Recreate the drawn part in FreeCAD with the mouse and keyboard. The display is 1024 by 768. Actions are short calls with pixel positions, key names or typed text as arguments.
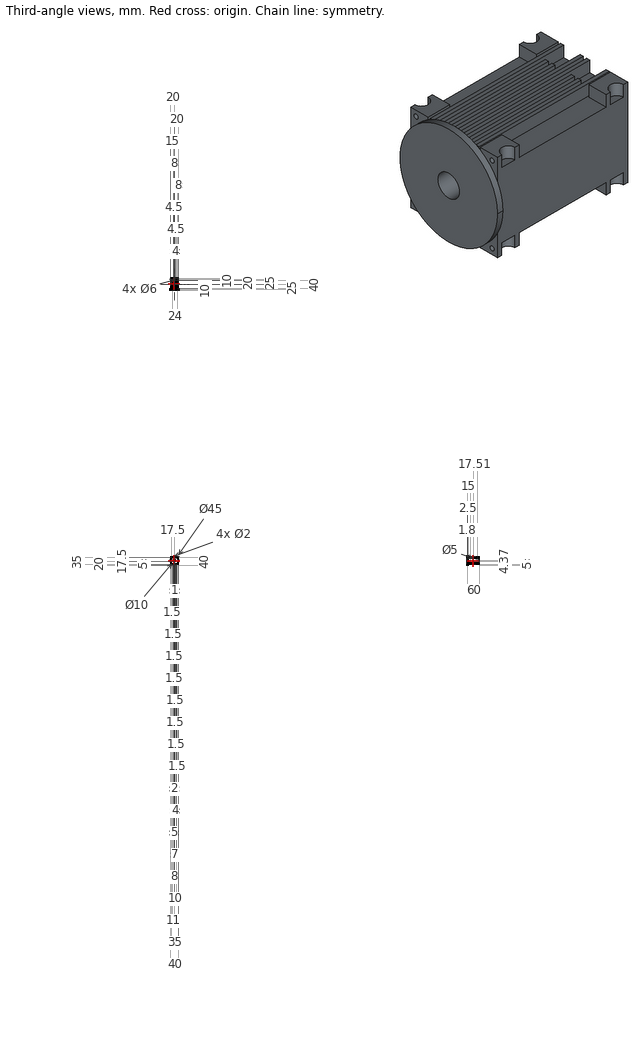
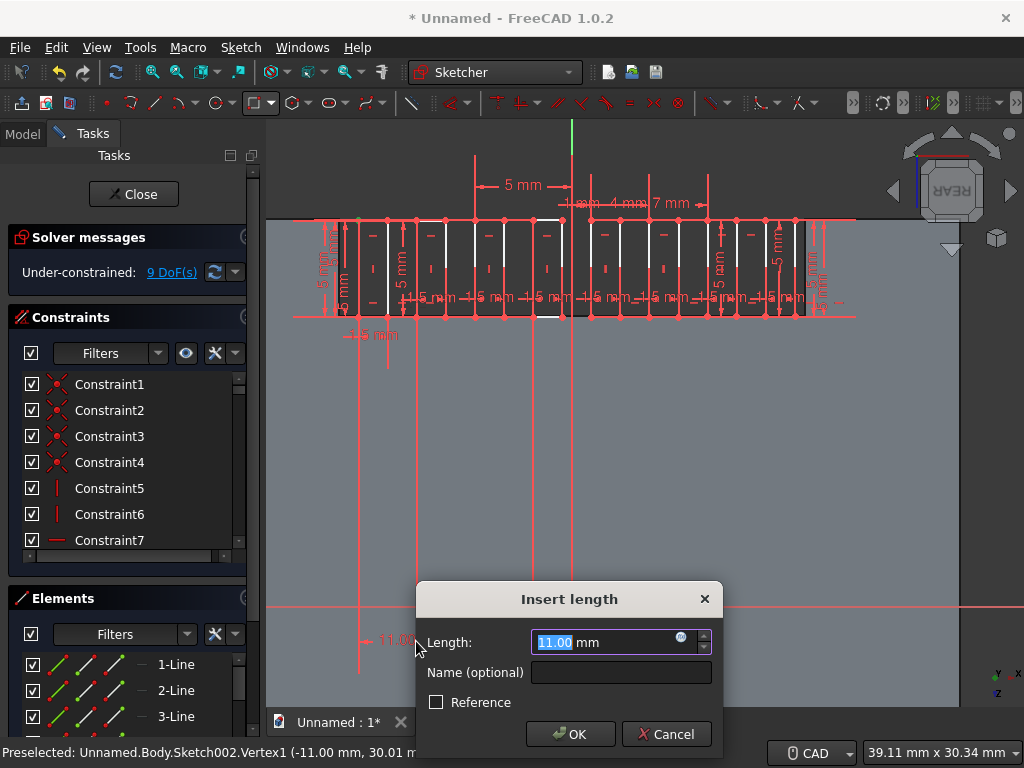
text(11)
key(Return)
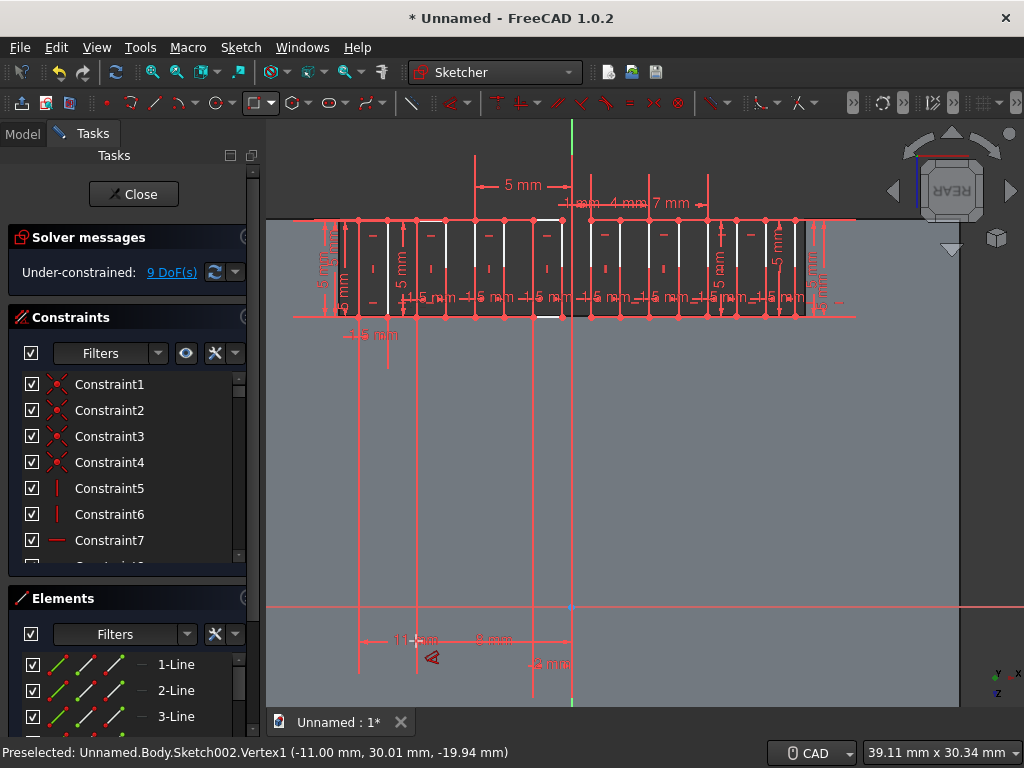
click(359, 221)
click(325, 414)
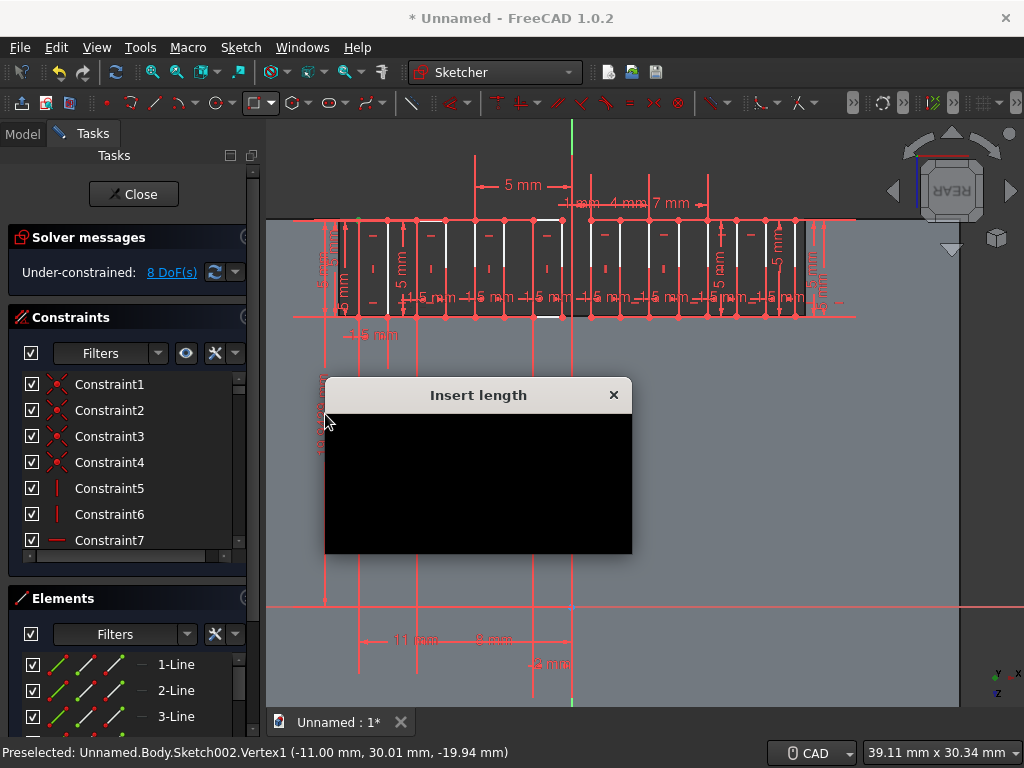
text(20)
key(Return)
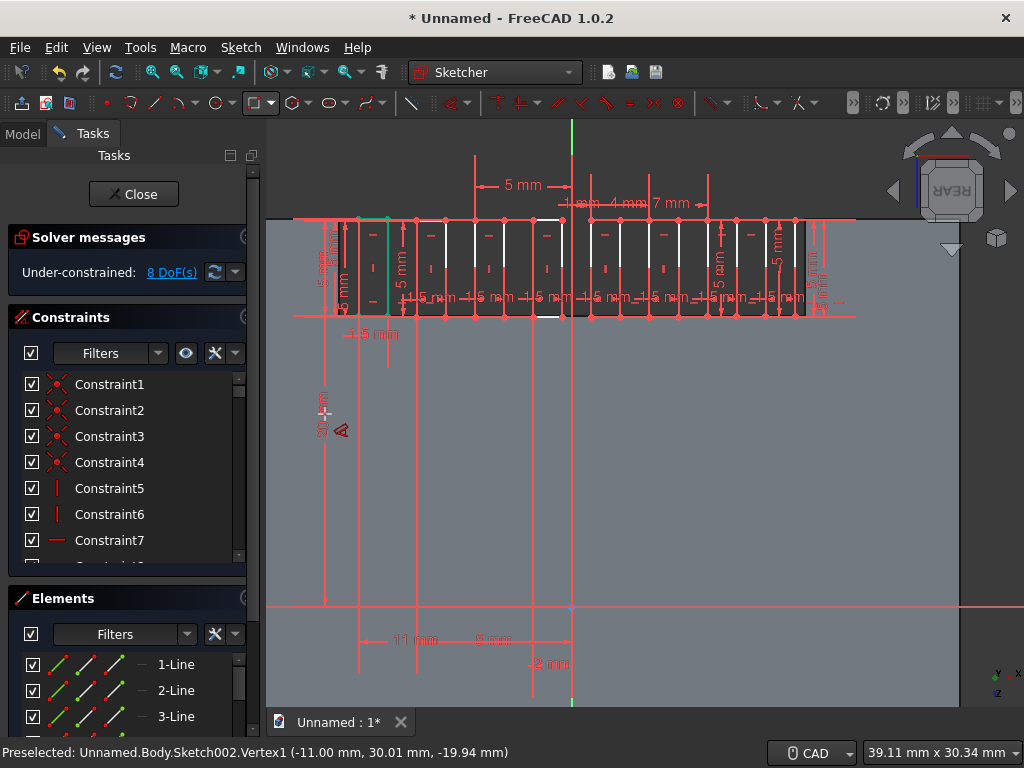
click(417, 221)
click(383, 503)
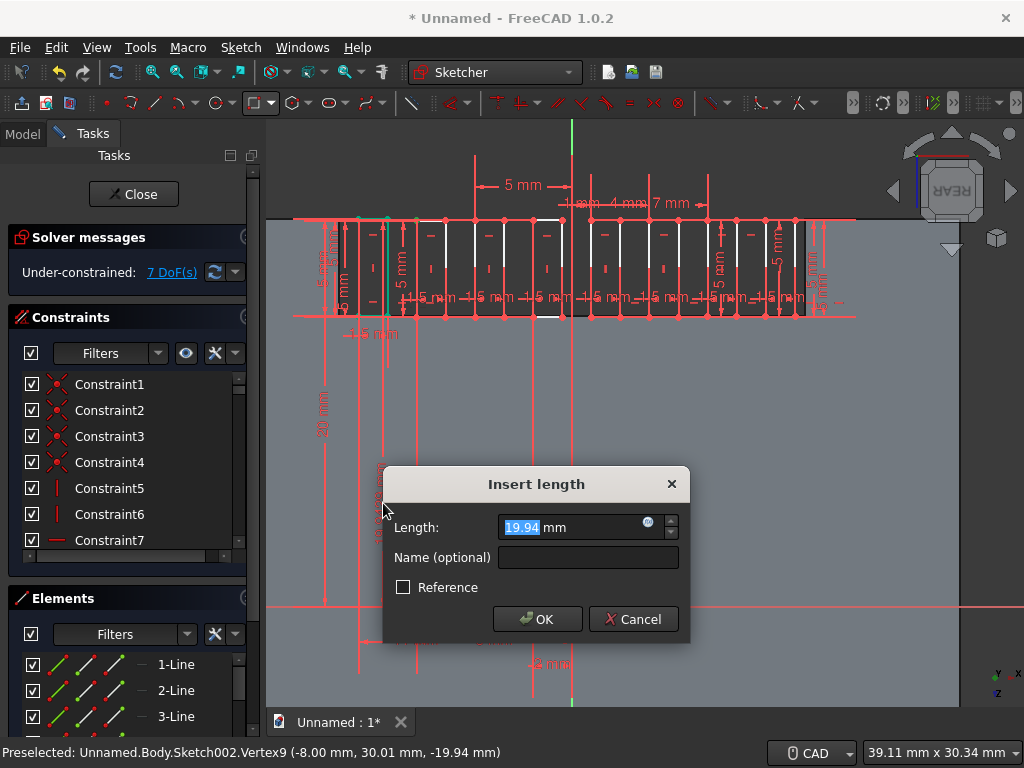
text(20)
key(Return)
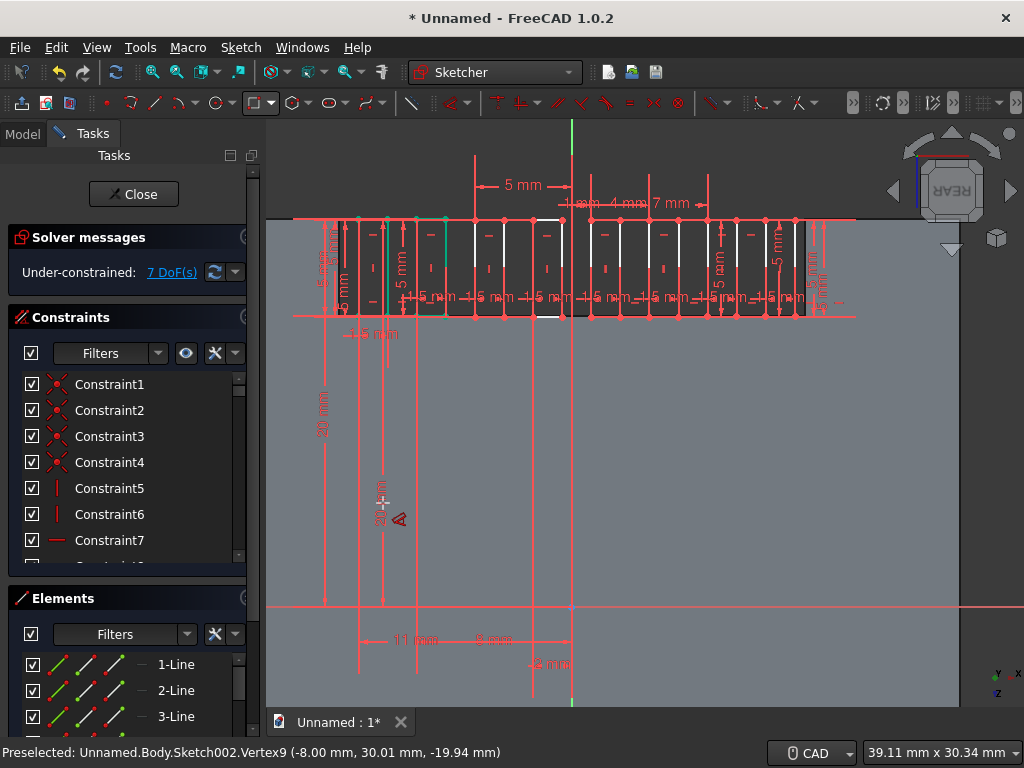
click(475, 220)
click(441, 414)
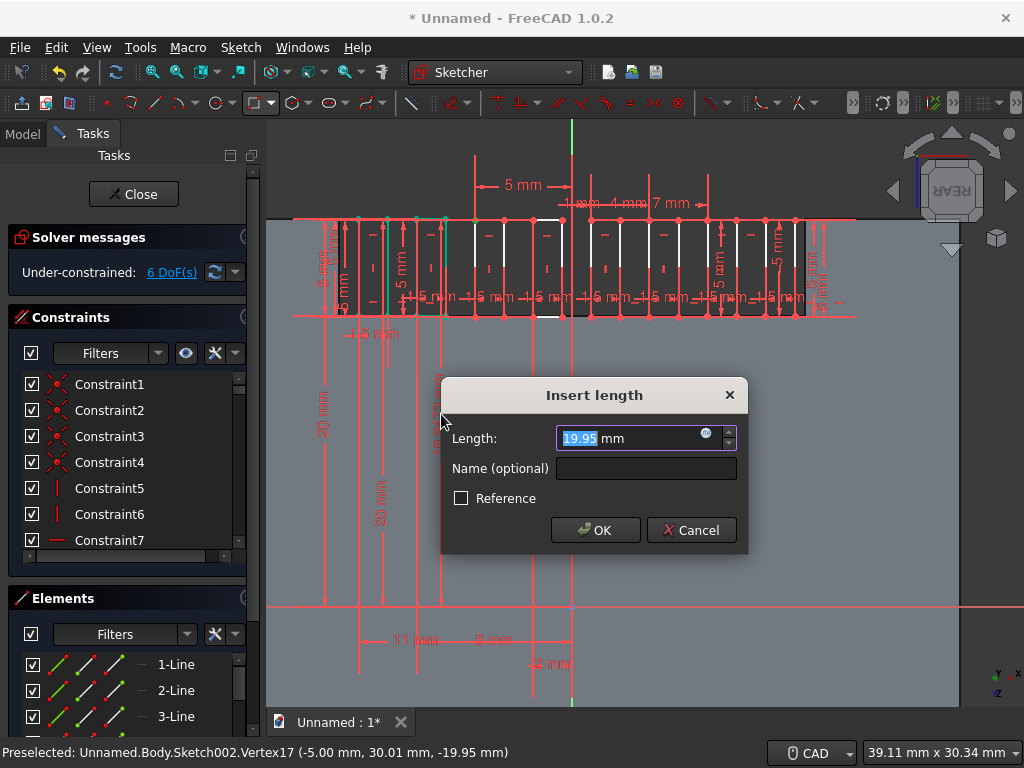
text(20)
key(Return)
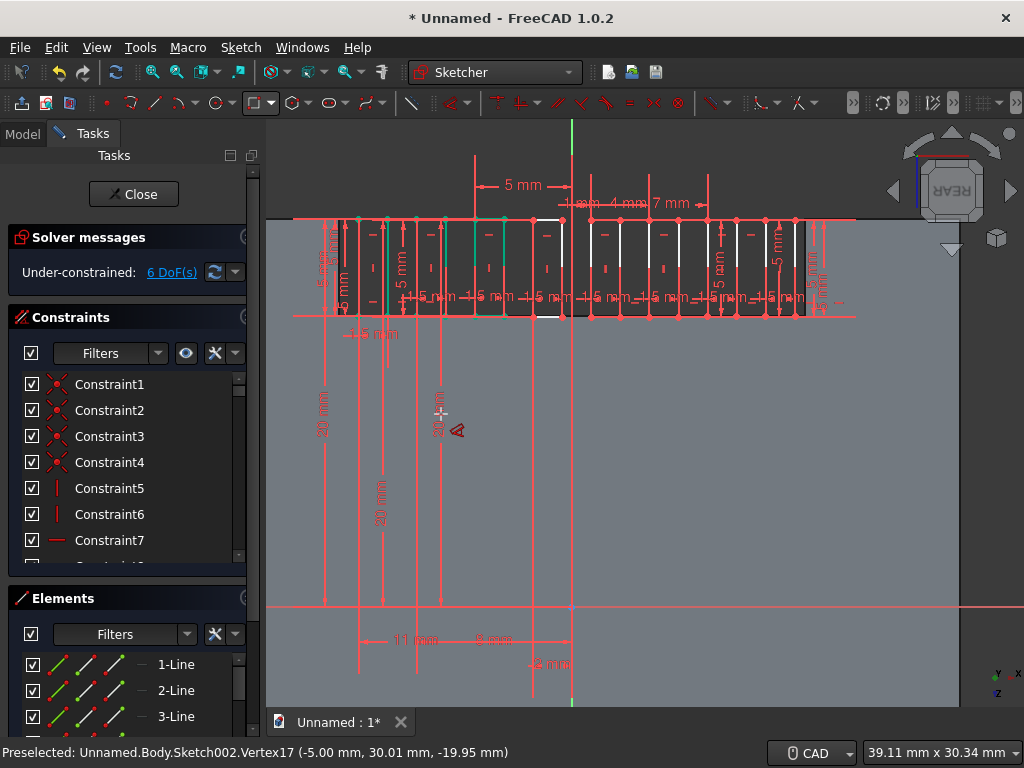
click(533, 220)
click(499, 503)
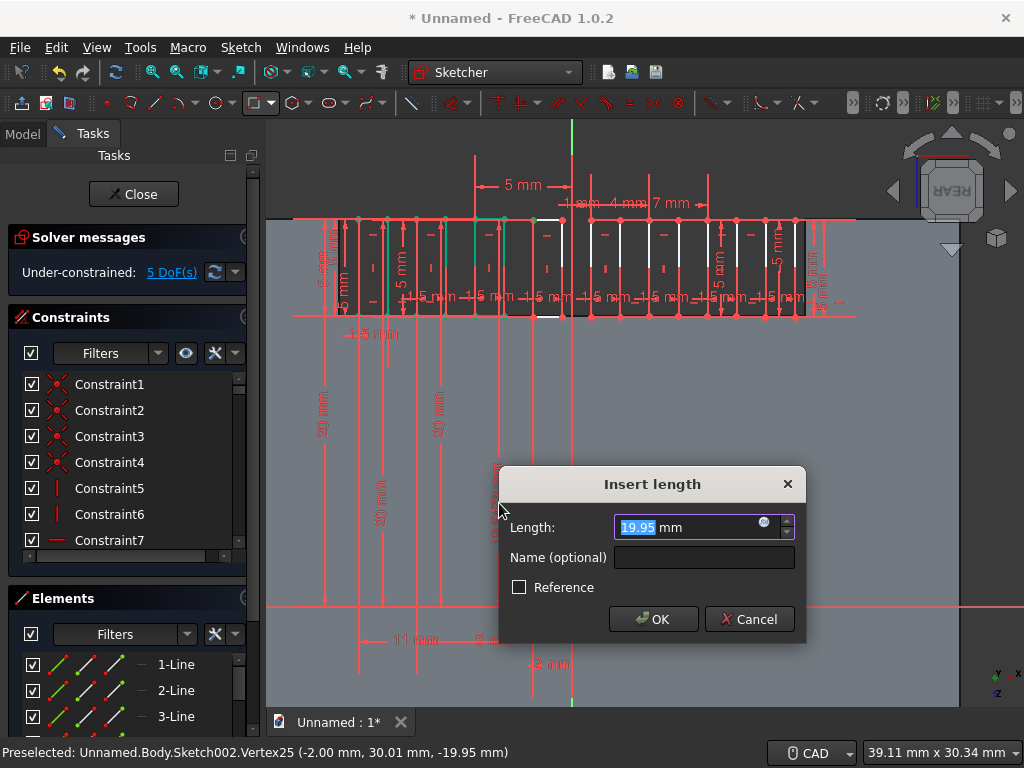
text(20)
key(Return)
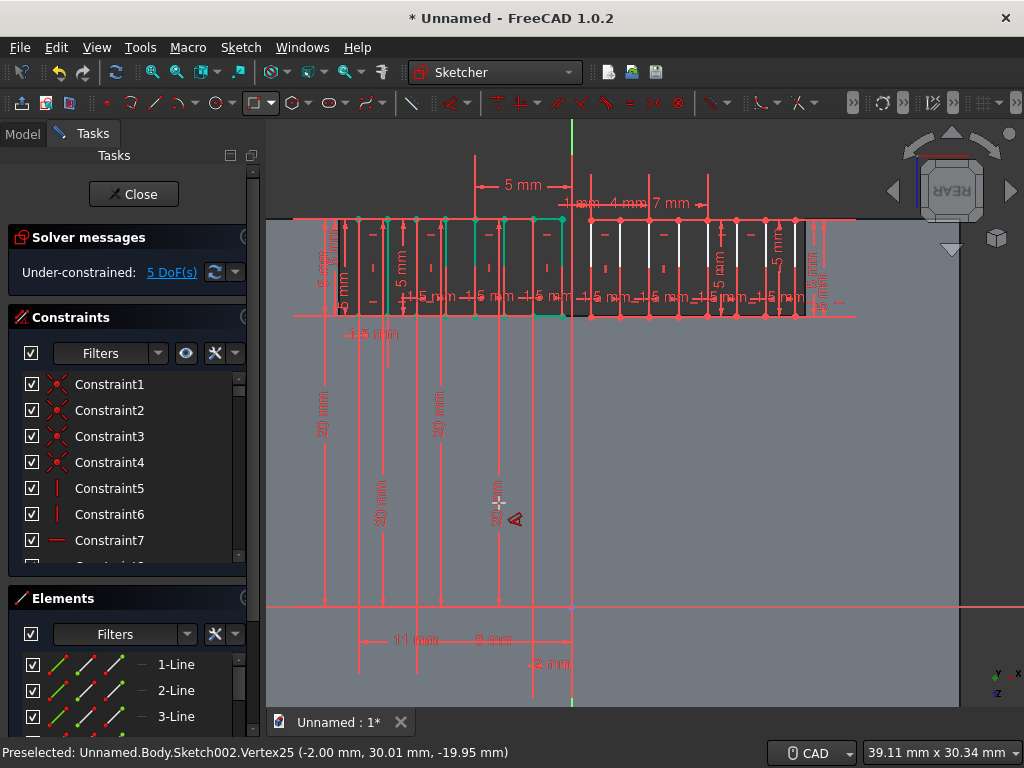
click(591, 220)
click(625, 414)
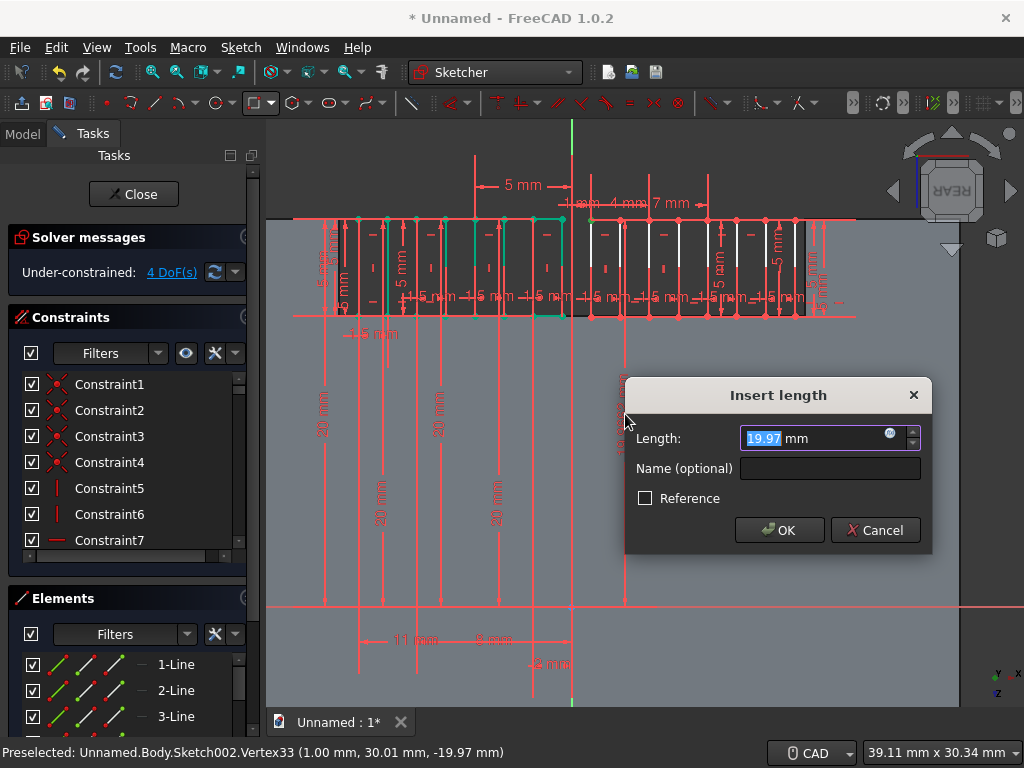
text(20)
key(Return)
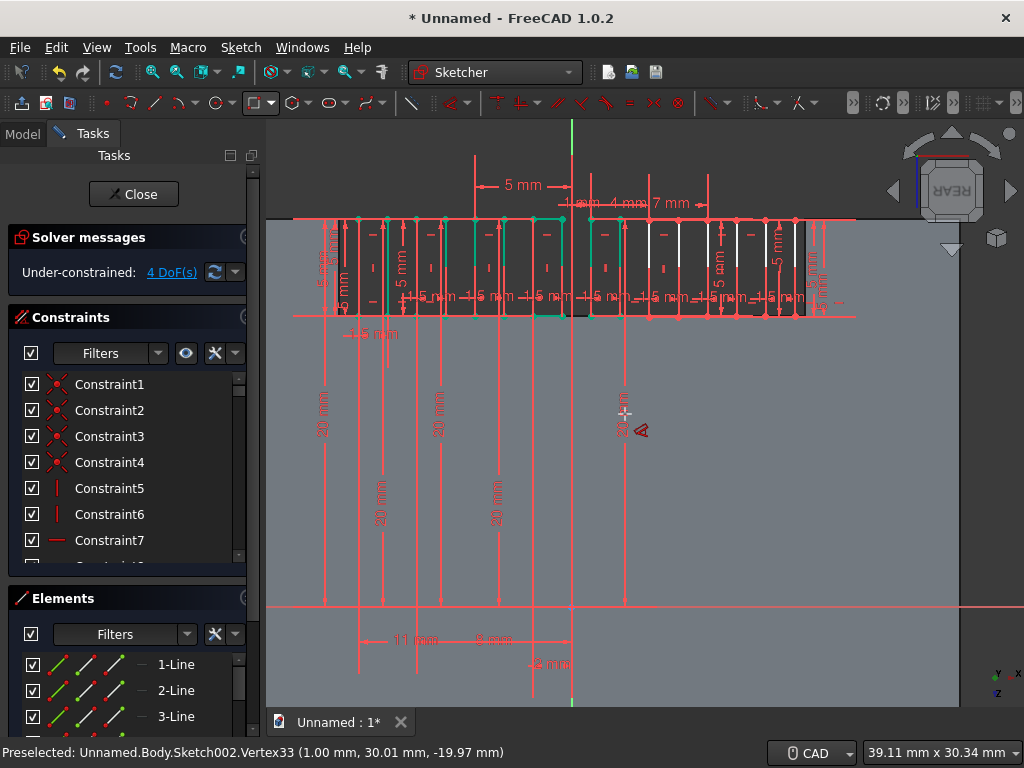
click(649, 220)
click(683, 503)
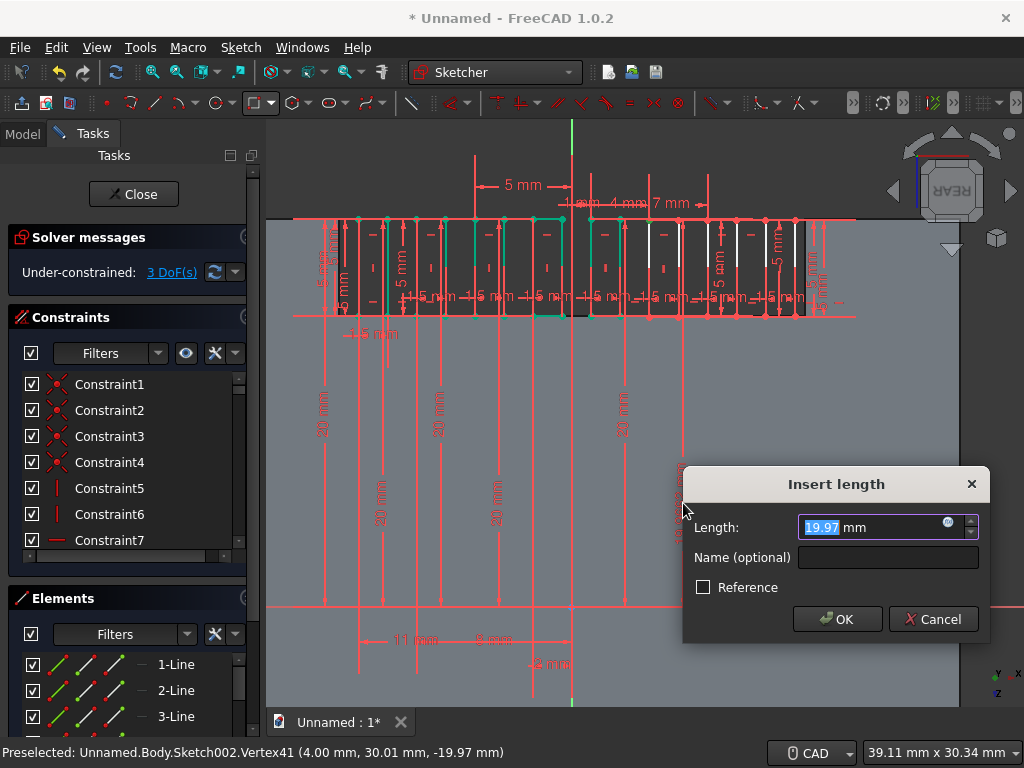
text(20)
key(Return)